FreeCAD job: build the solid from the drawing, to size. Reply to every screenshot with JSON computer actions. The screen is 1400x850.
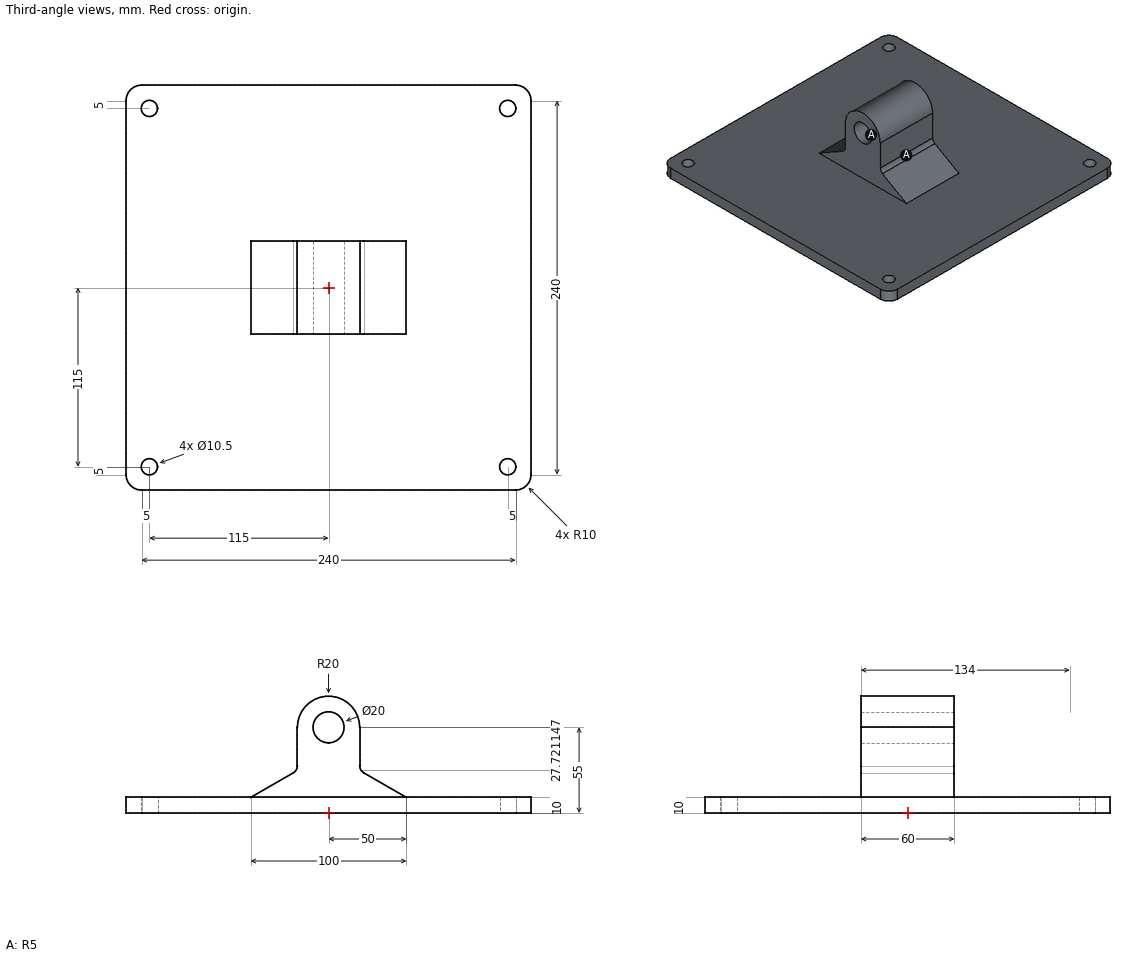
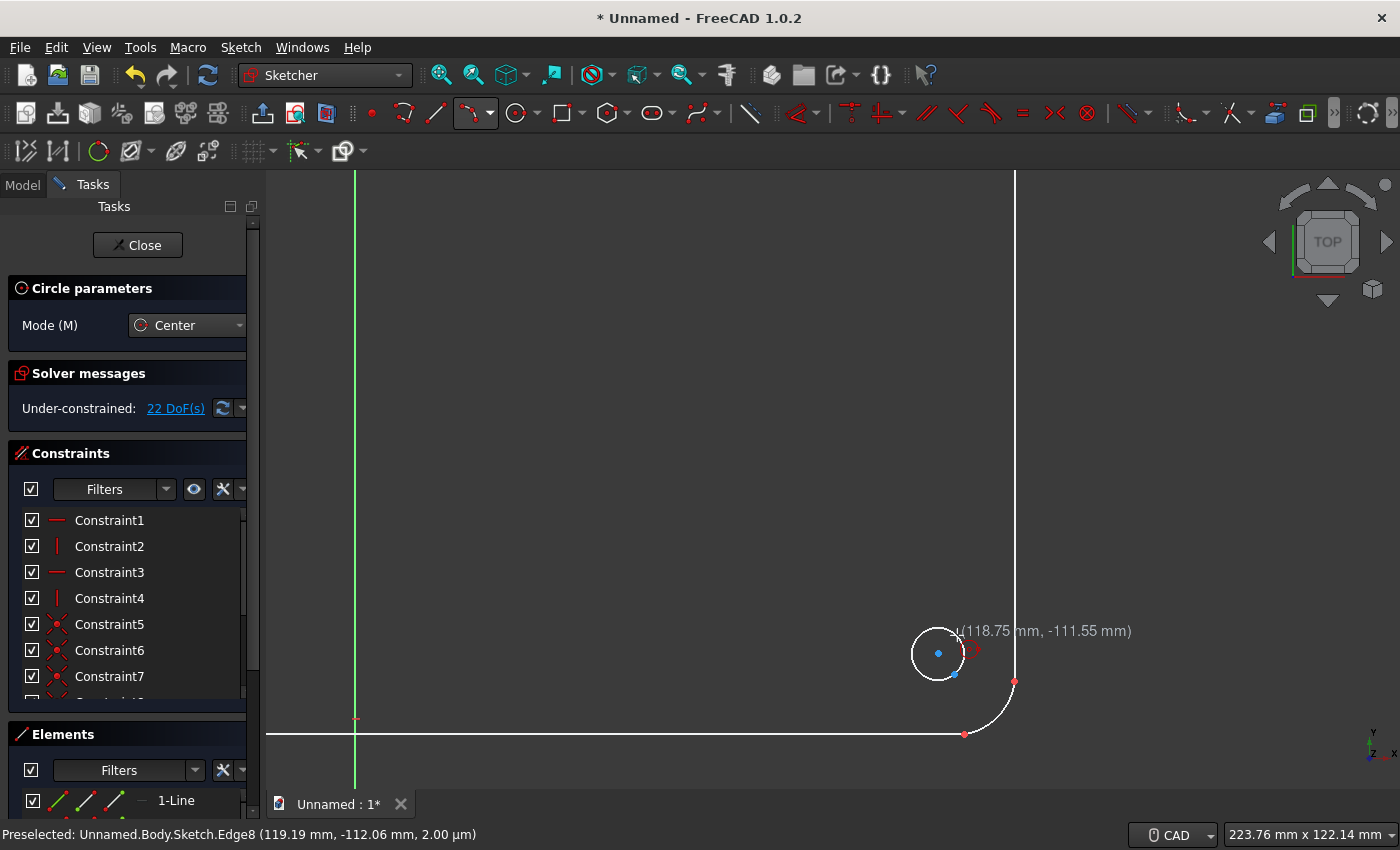
{"action": "scroll", "coordinate": [941, 656], "scroll_direction": "down", "scroll_amount": 6}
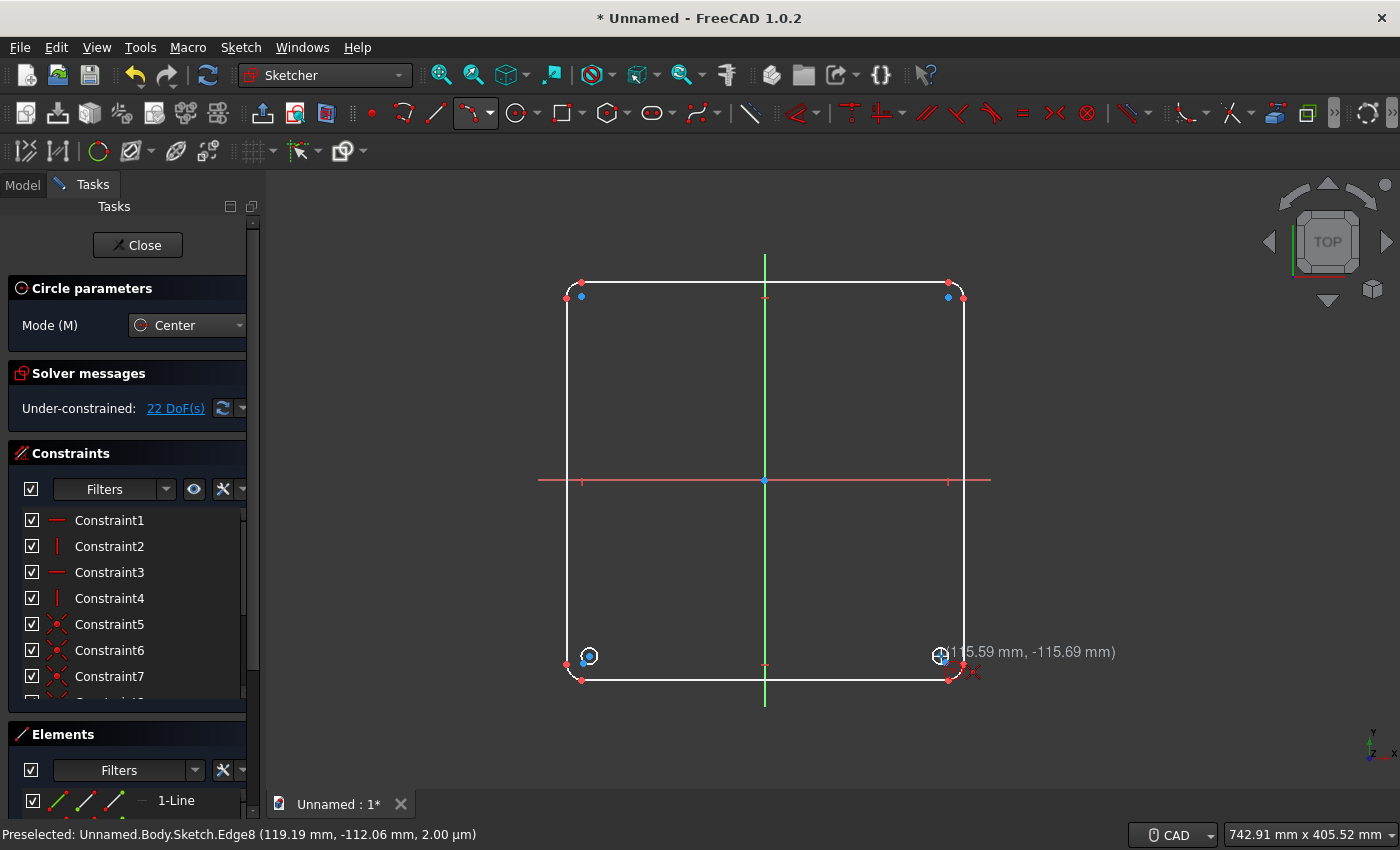
{"action": "scroll", "coordinate": [589, 305], "scroll_direction": "up", "scroll_amount": 6}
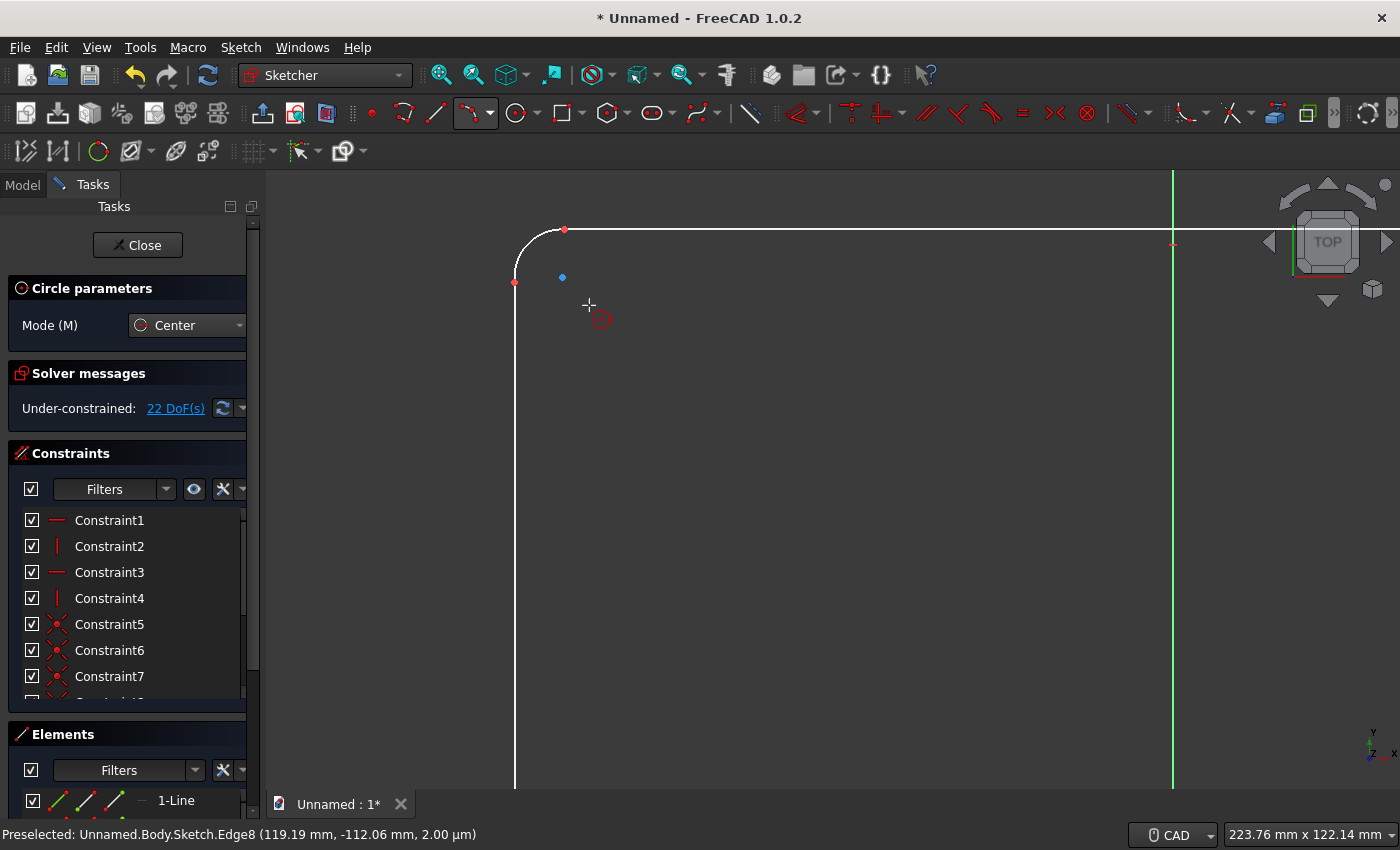
{"action": "left_click", "coordinate": [590, 304]}
{"action": "left_click", "coordinate": [609, 285]}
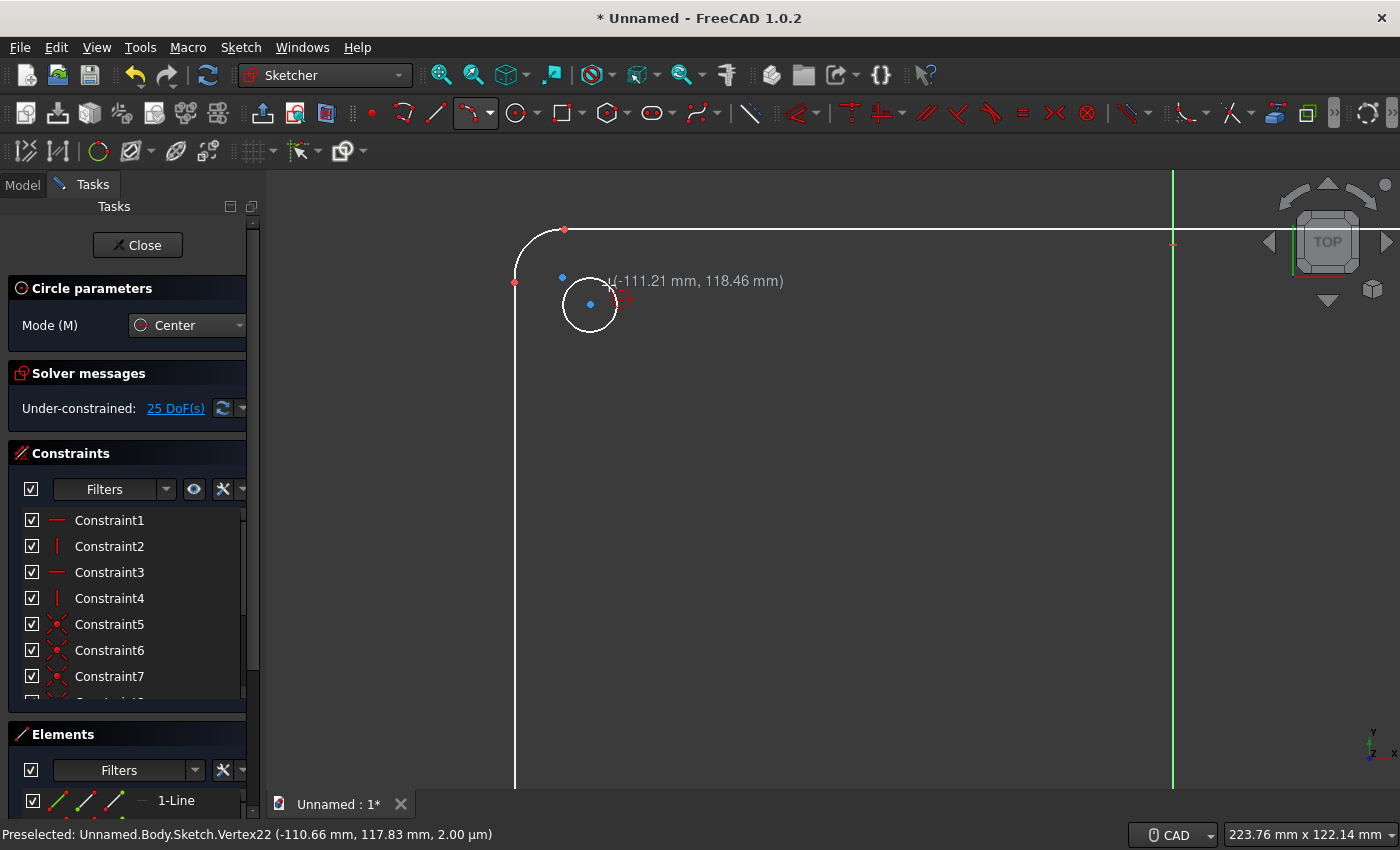
{"action": "scroll", "coordinate": [589, 304], "scroll_direction": "down", "scroll_amount": 6}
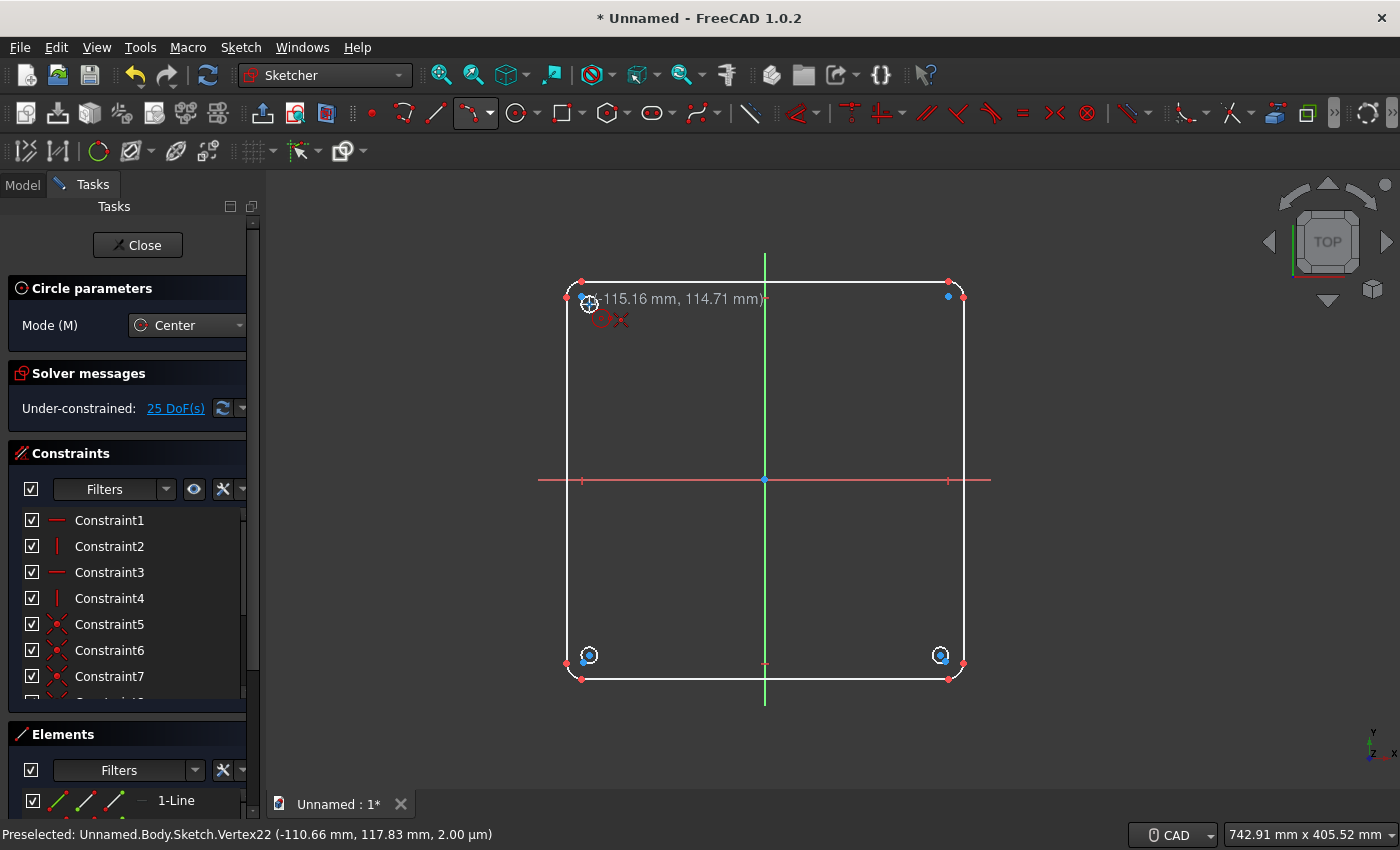
{"action": "scroll", "coordinate": [941, 304], "scroll_direction": "up", "scroll_amount": 6}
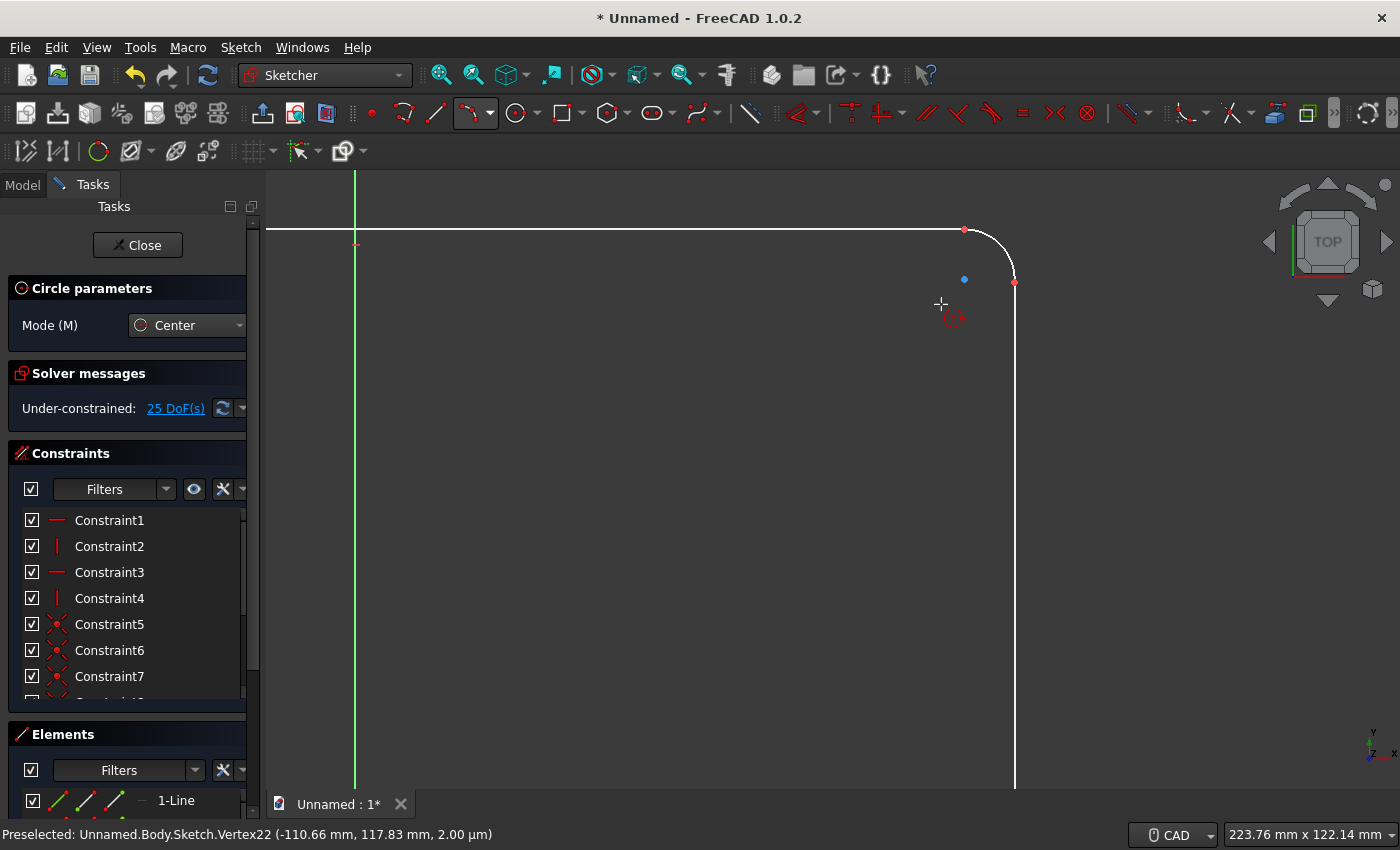
{"action": "left_click", "coordinate": [938, 304]}
{"action": "left_click", "coordinate": [919, 285]}
{"action": "key", "text": "Escape"}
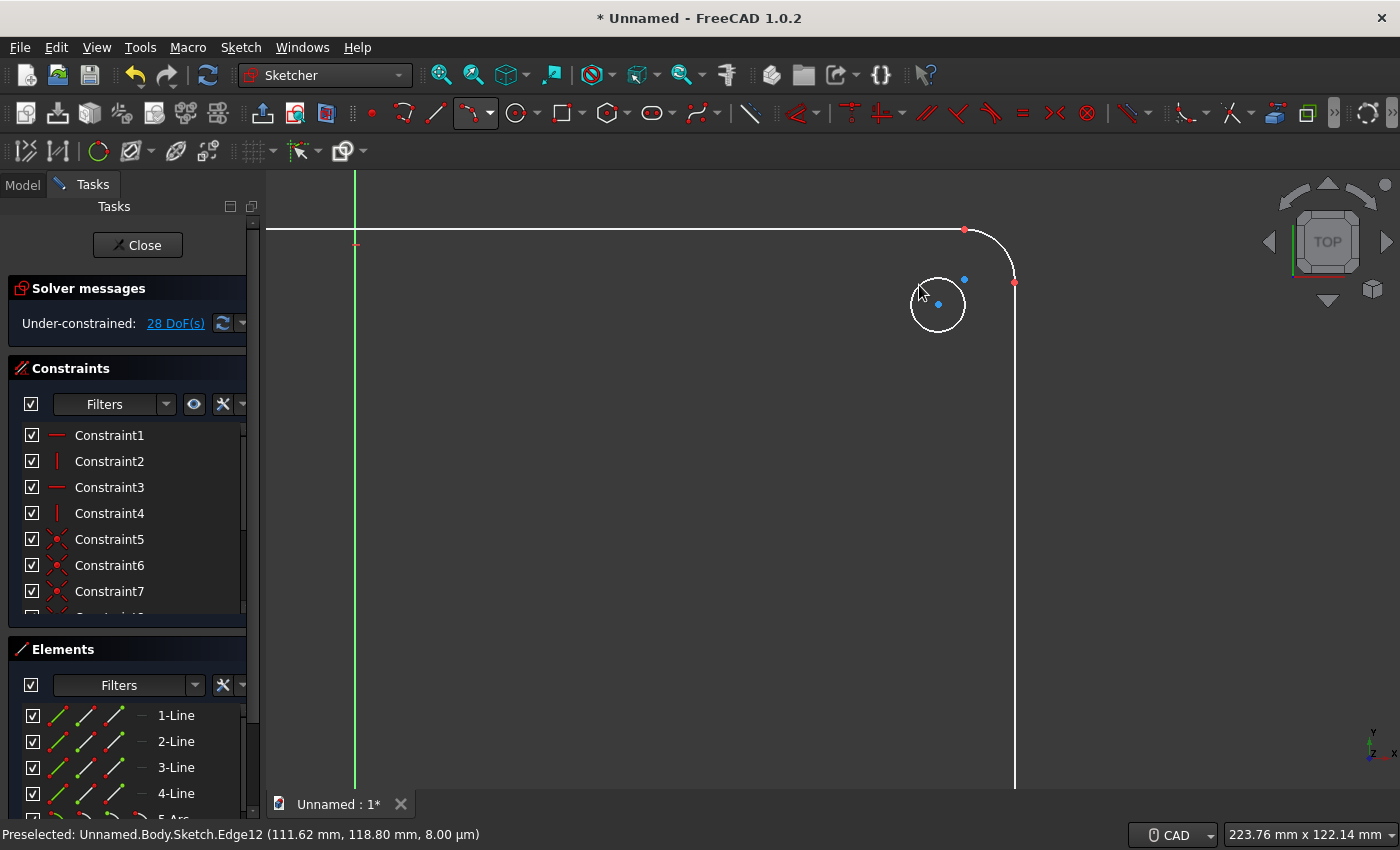
{"action": "scroll", "coordinate": [941, 304], "scroll_direction": "down", "scroll_amount": 6}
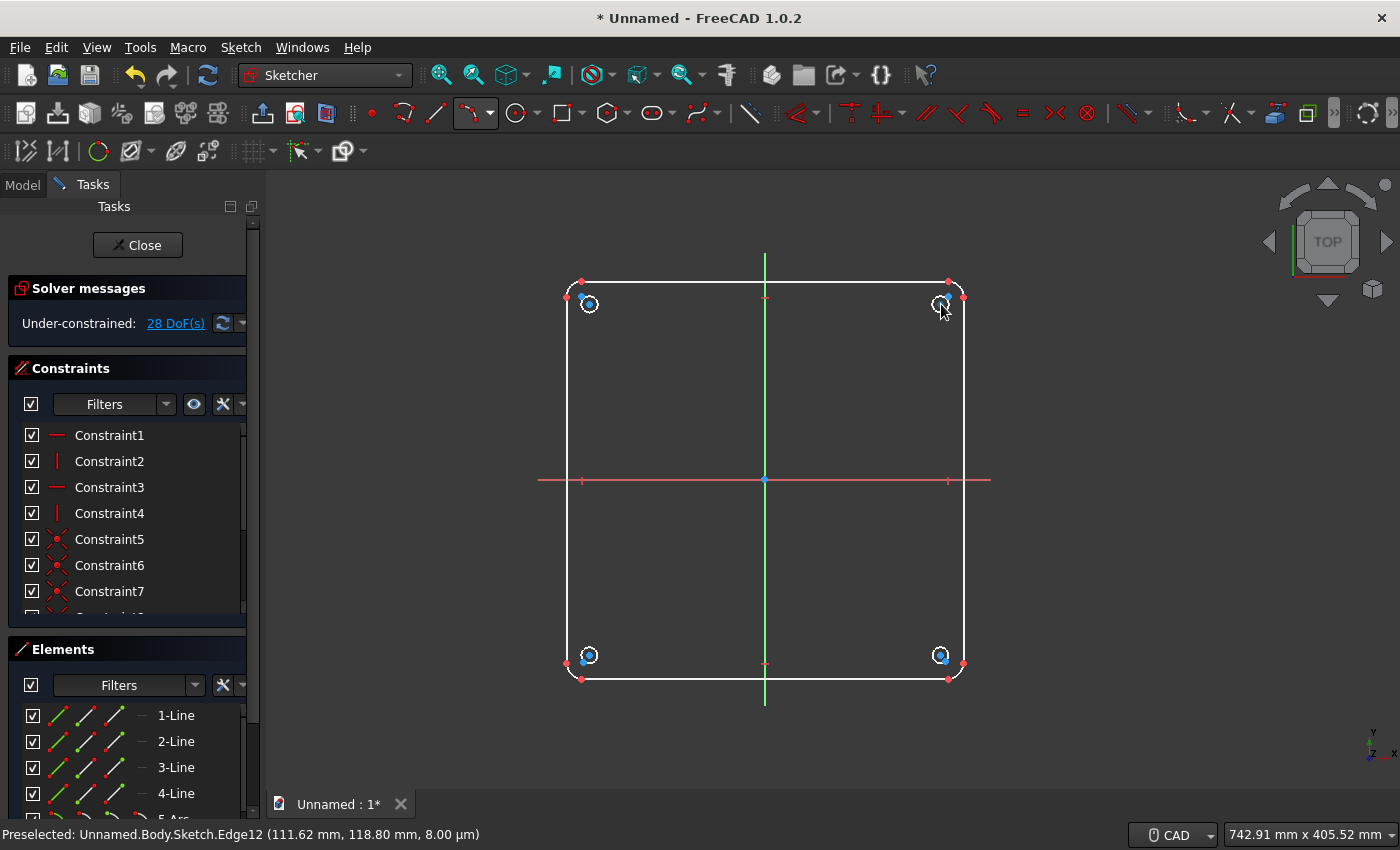
{"action": "left_click", "coordinate": [692, 679]}